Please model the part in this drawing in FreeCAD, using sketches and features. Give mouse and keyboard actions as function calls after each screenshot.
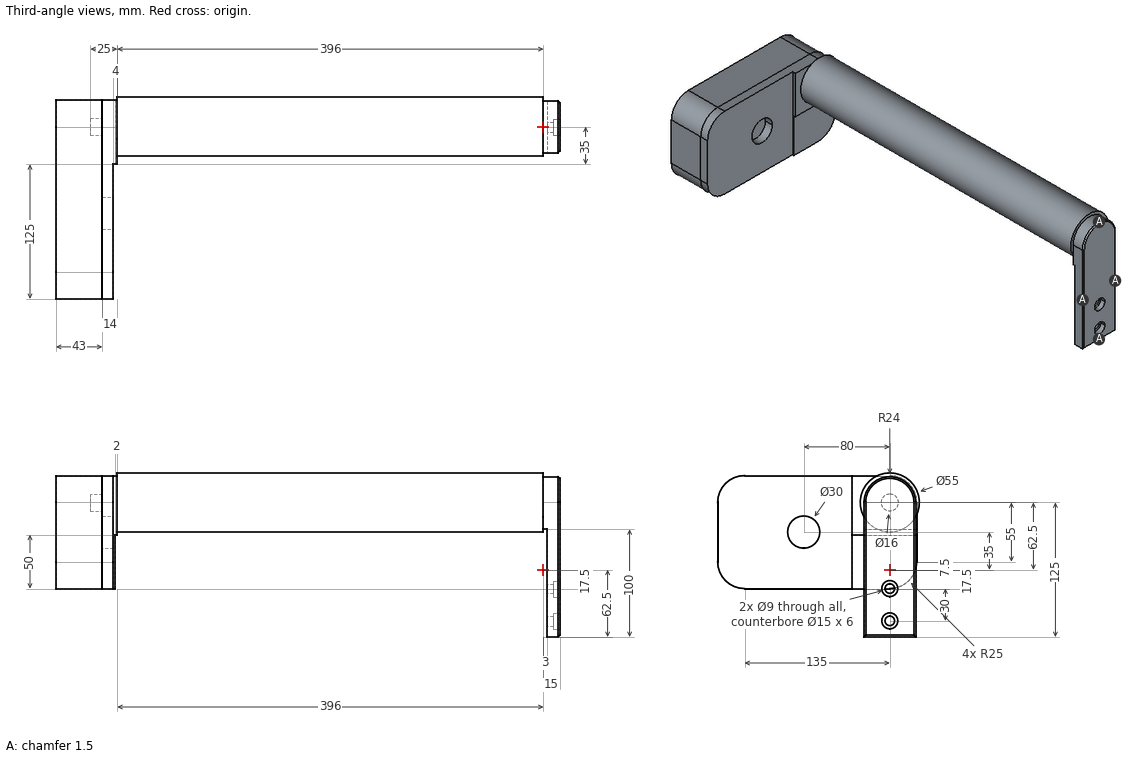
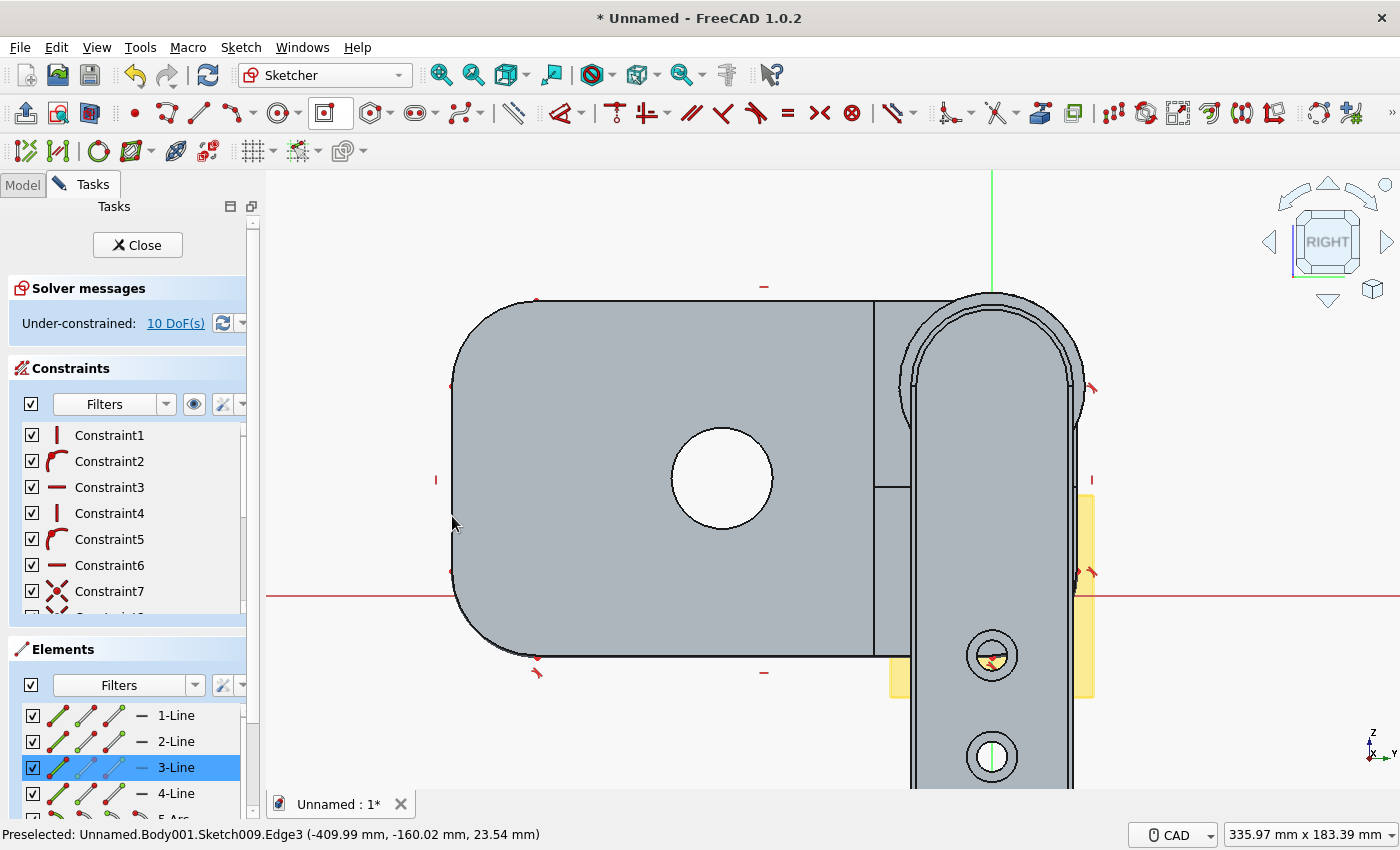
click(461, 611)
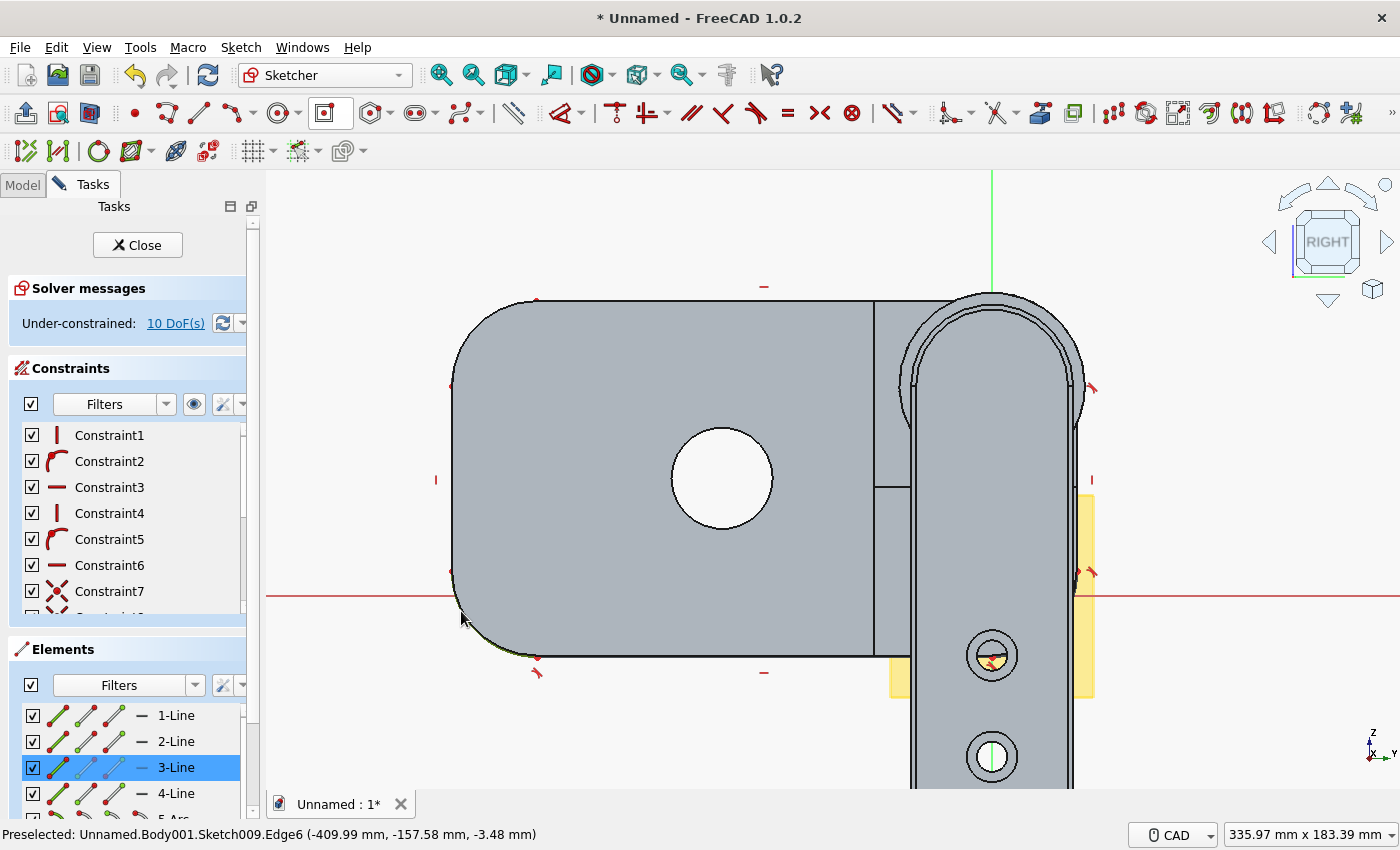
key(t)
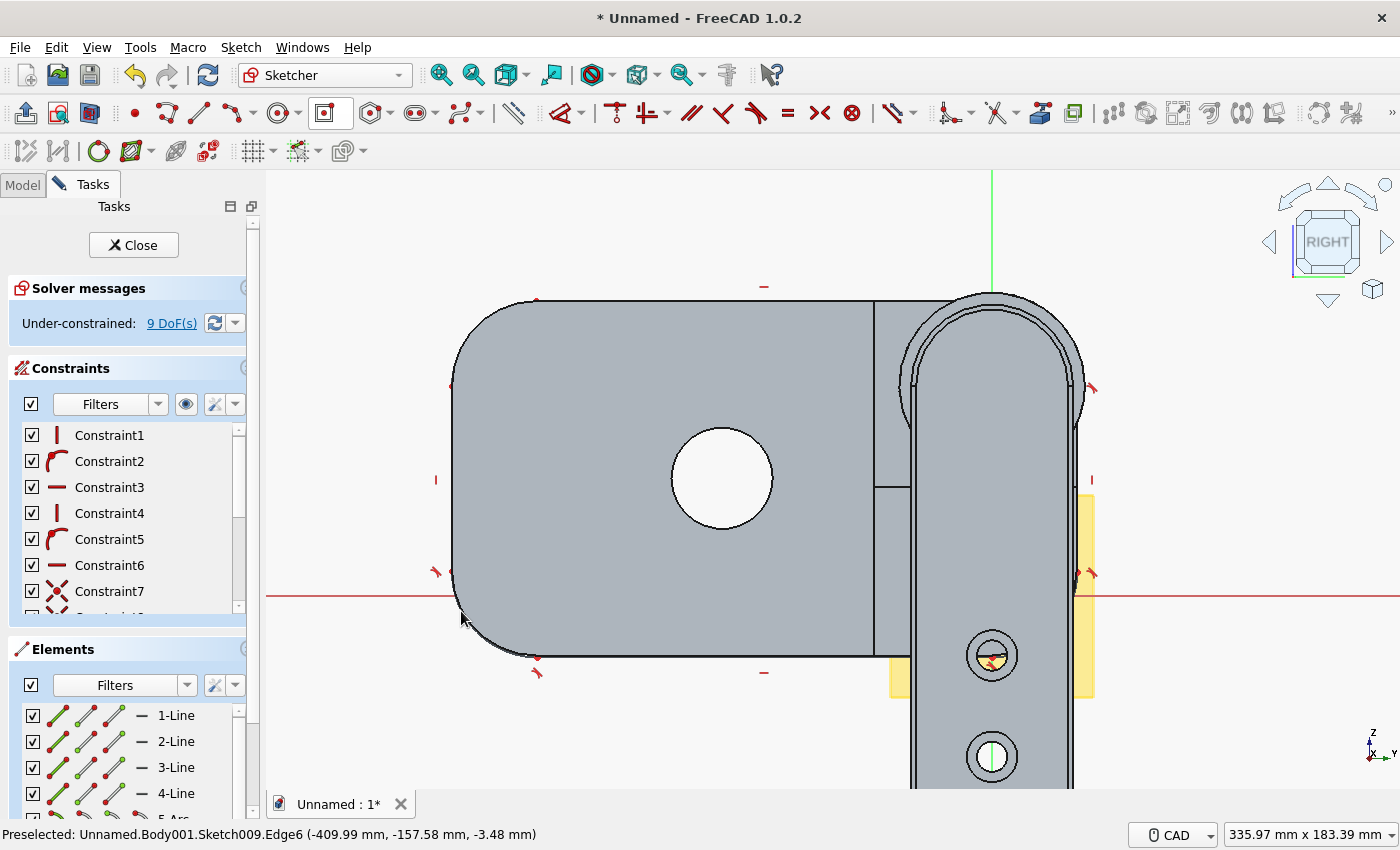
click(452, 516)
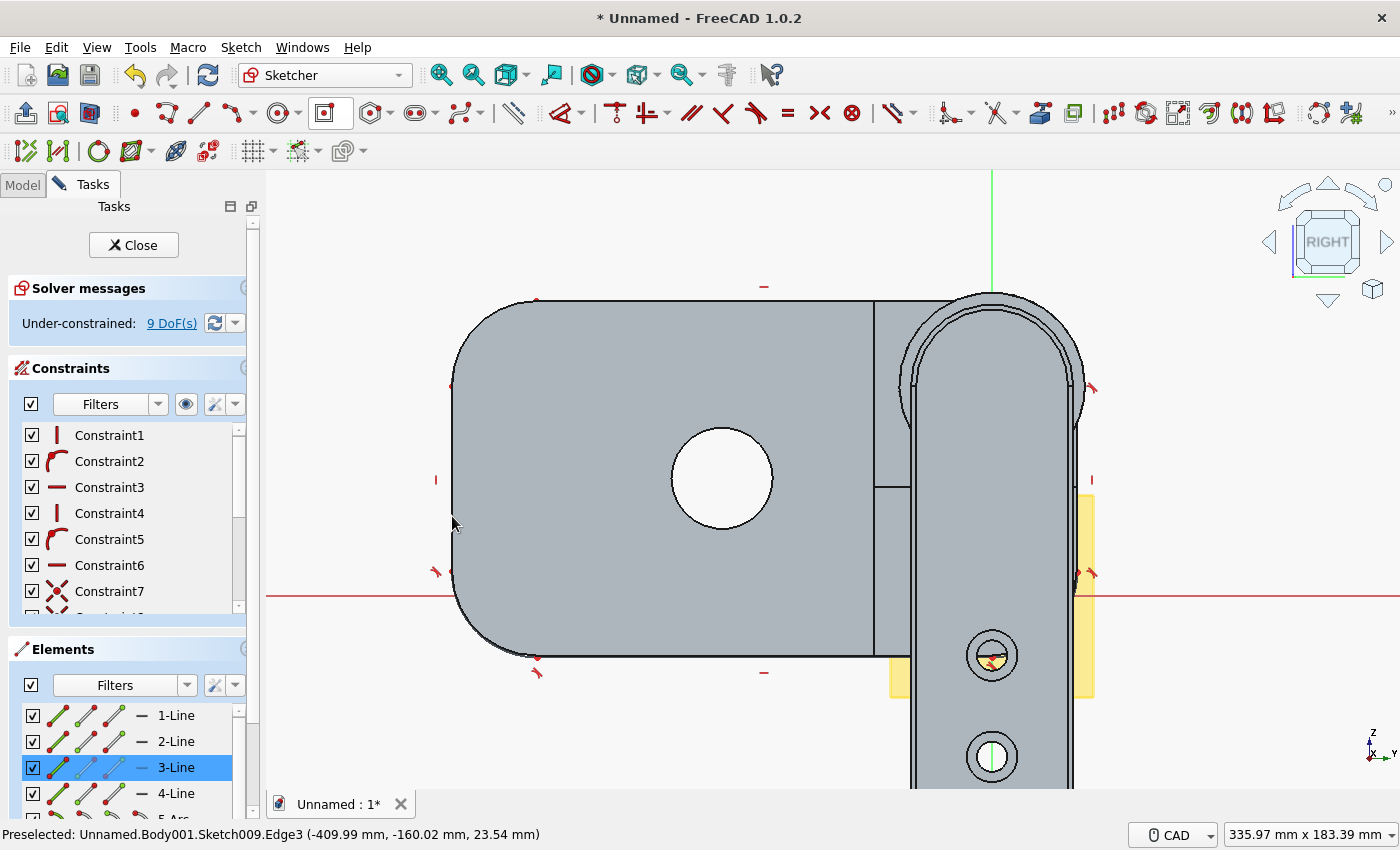
click(498, 312)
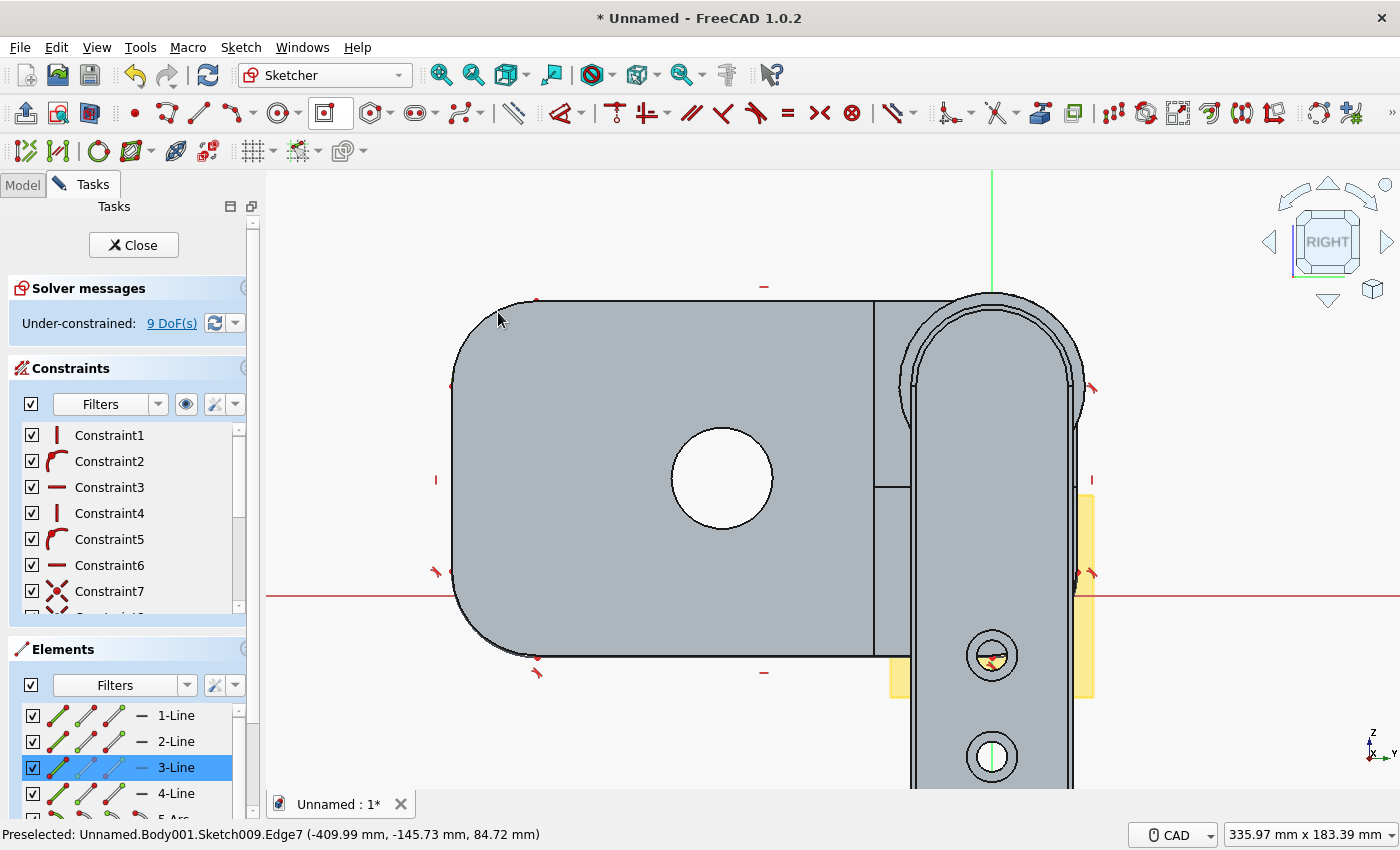
click(756, 114)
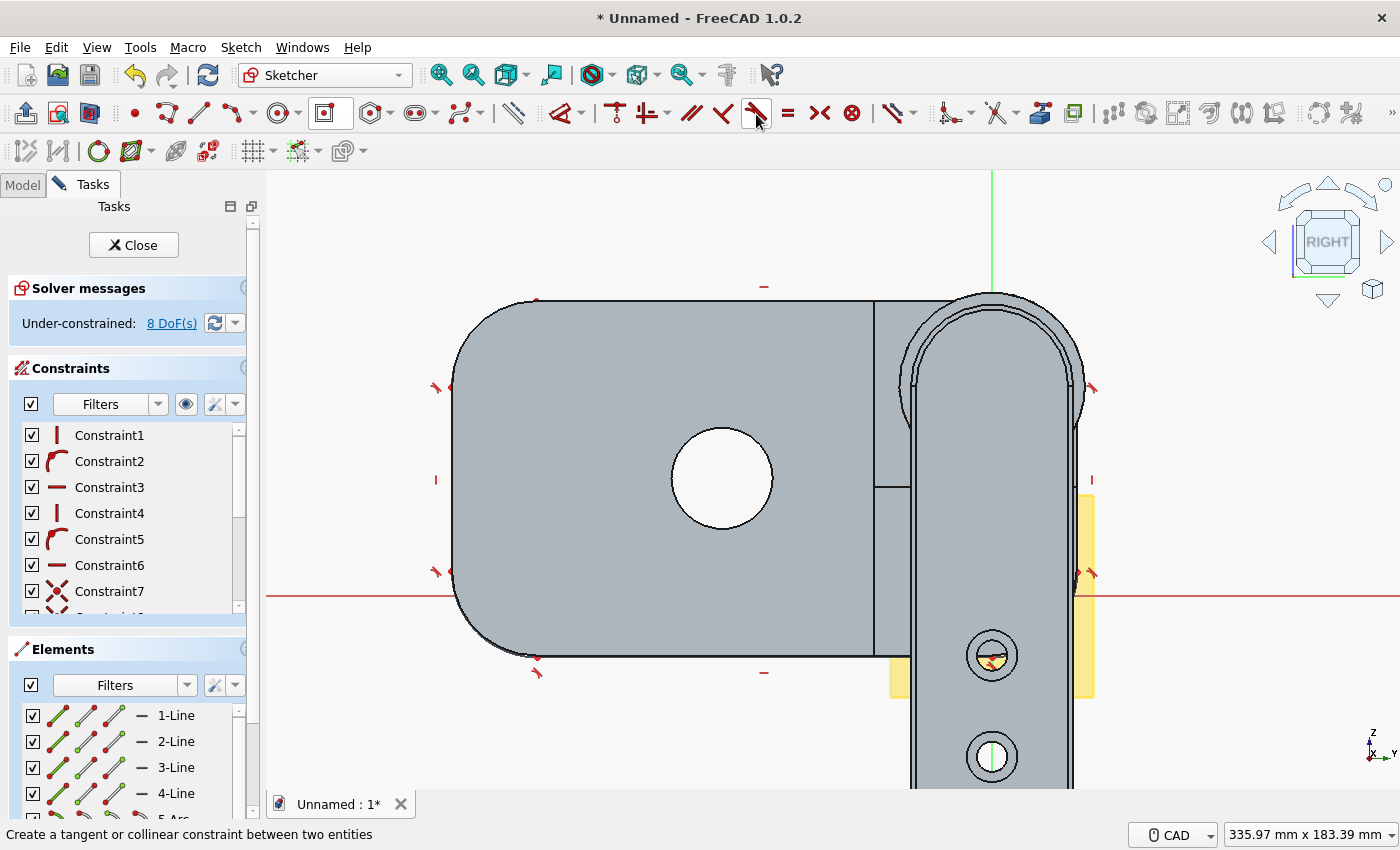
click(673, 302)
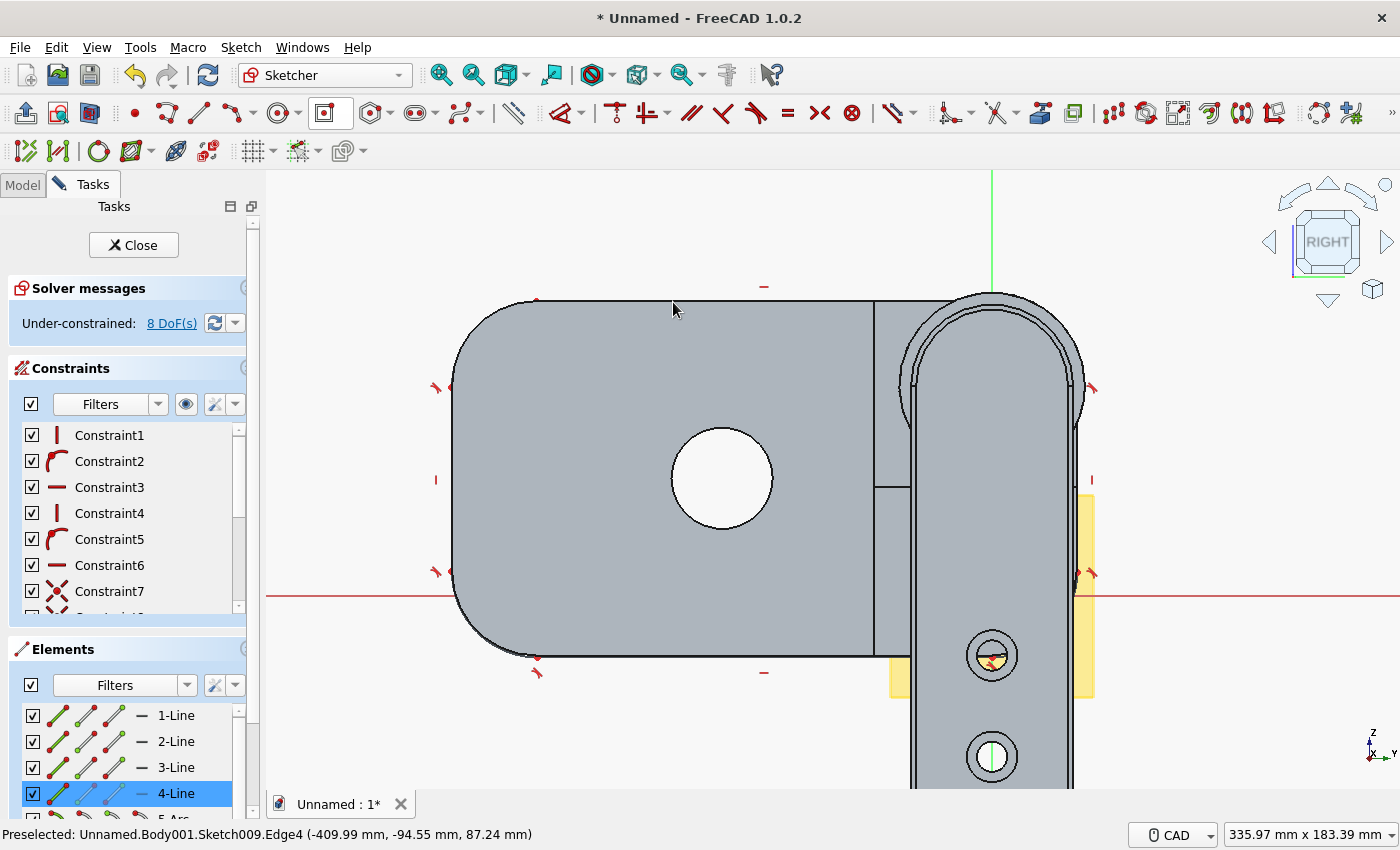
click(498, 312)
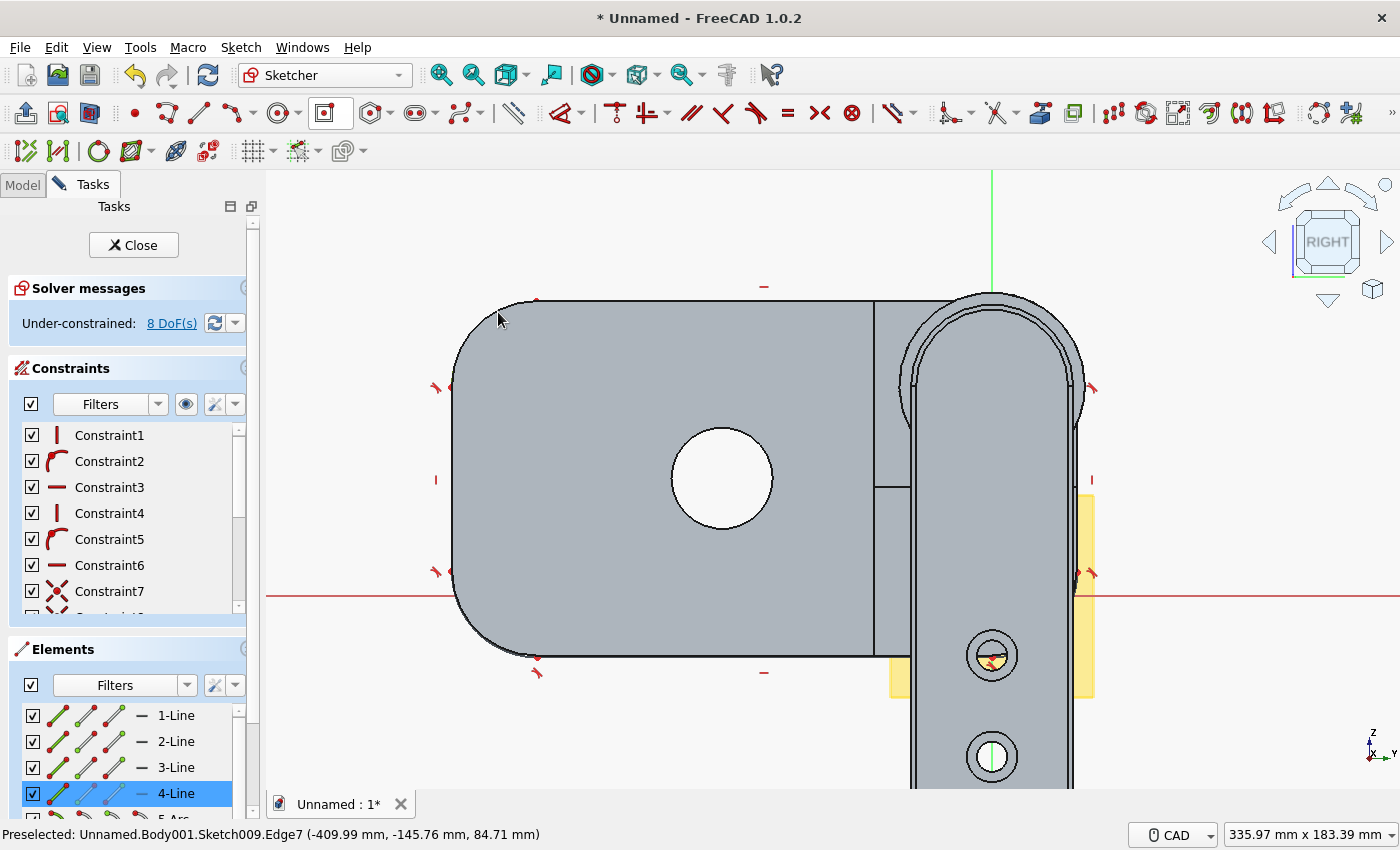
key(t)